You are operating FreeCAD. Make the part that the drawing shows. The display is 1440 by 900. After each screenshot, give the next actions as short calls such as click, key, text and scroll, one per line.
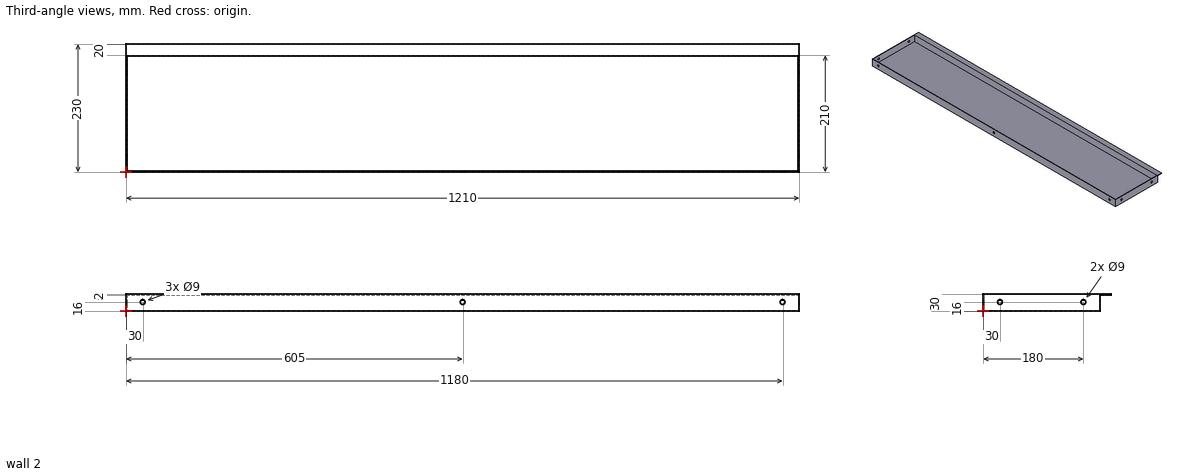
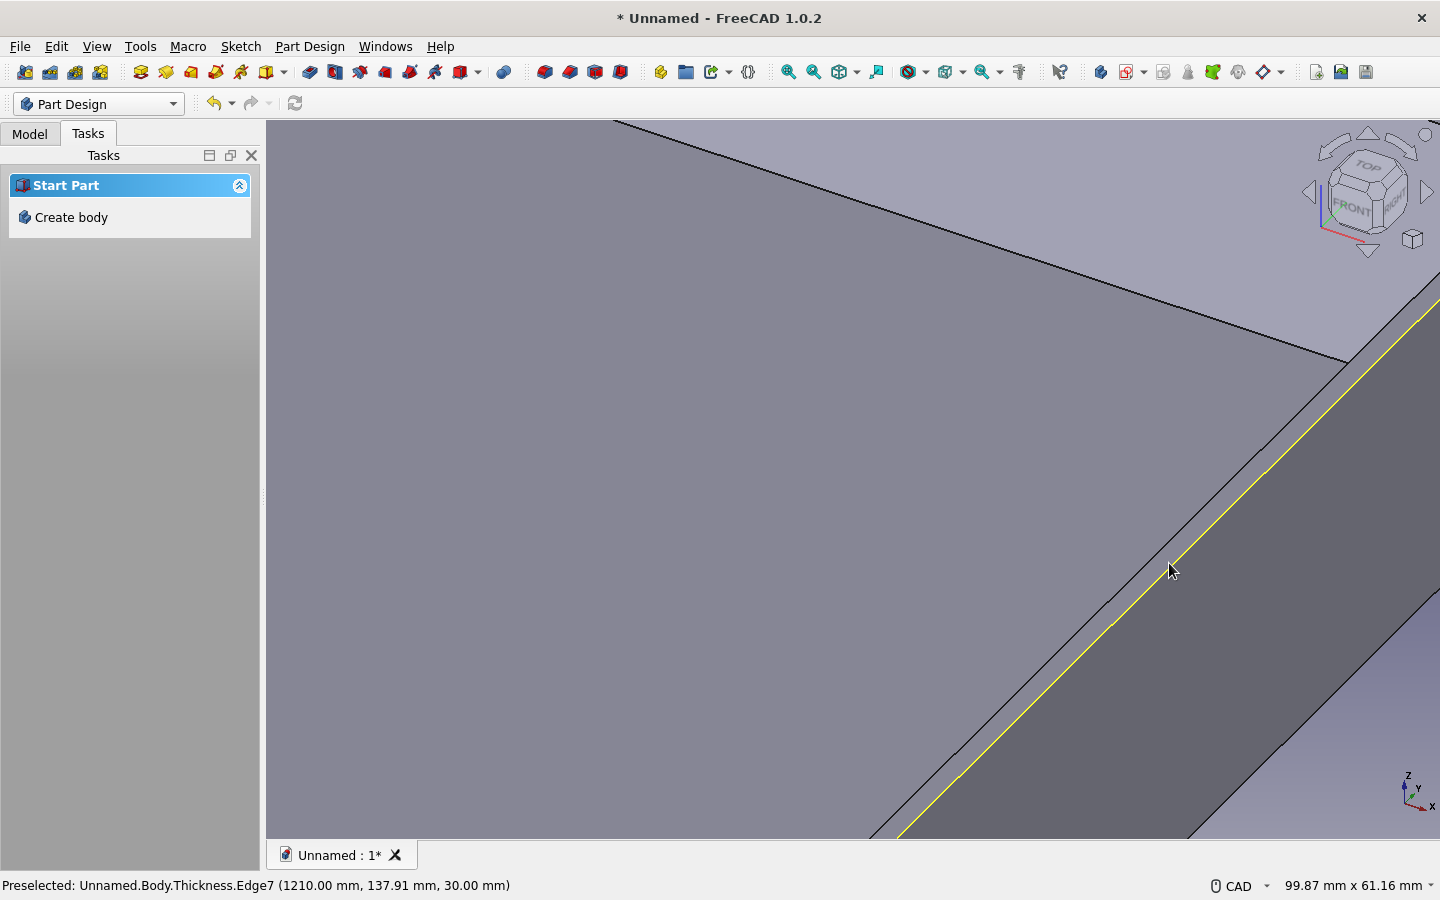
click(789, 72)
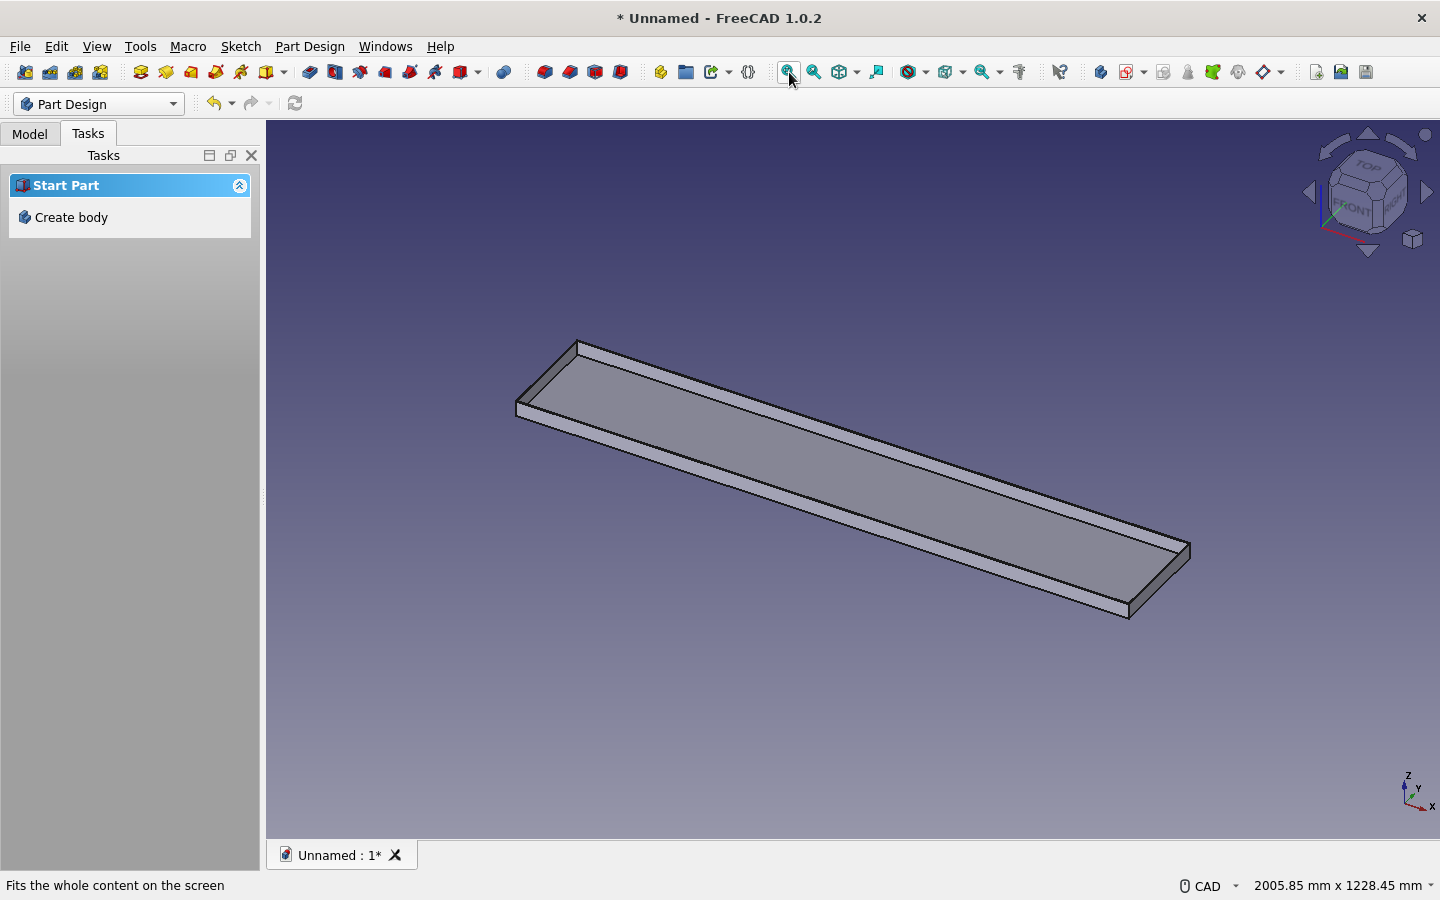
key(0)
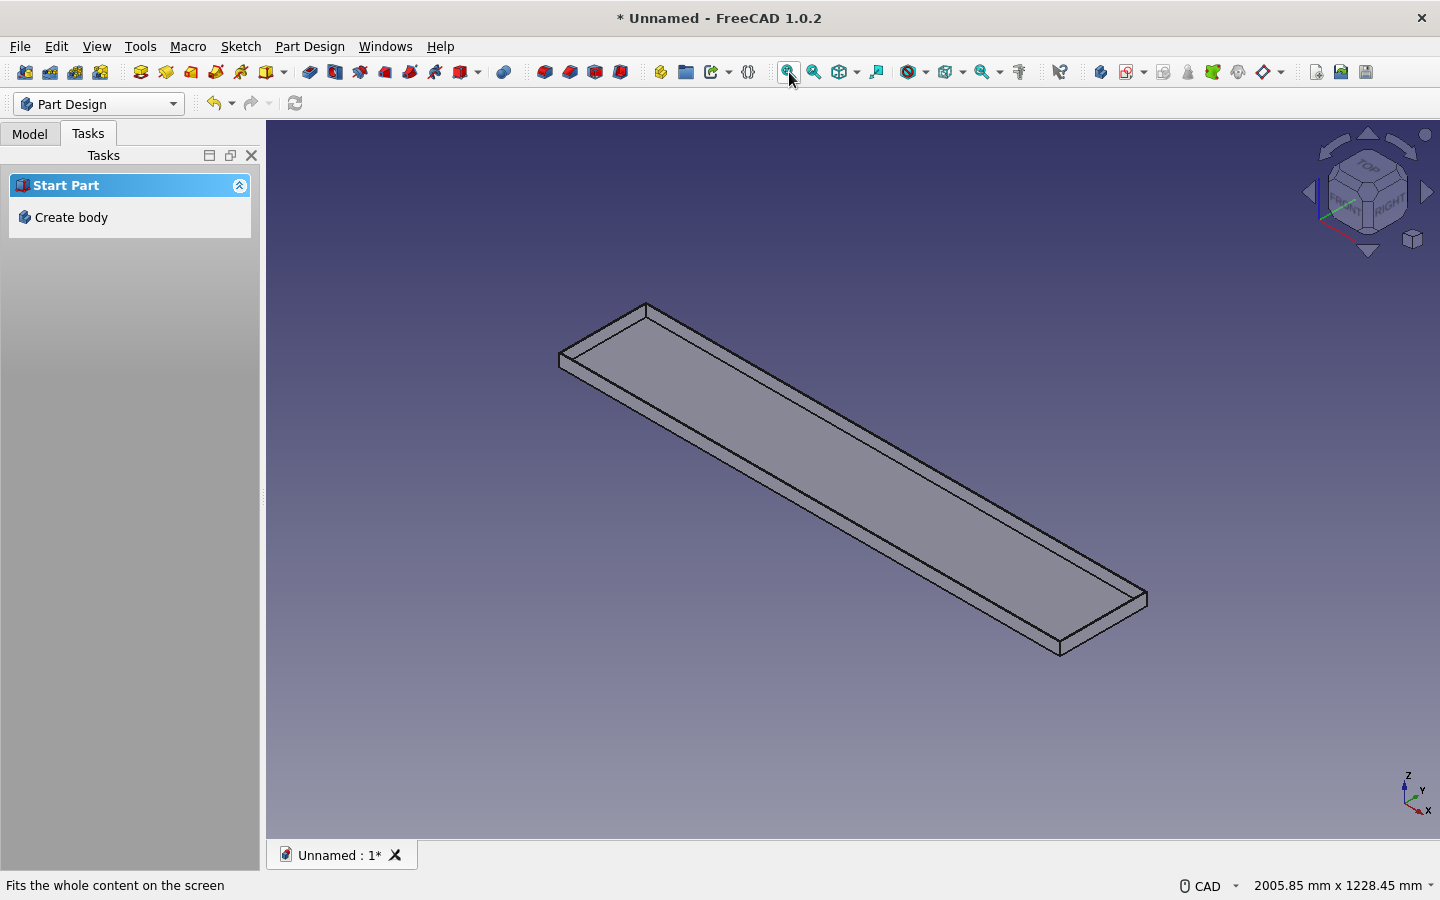
scroll(1117, 608, up, 15)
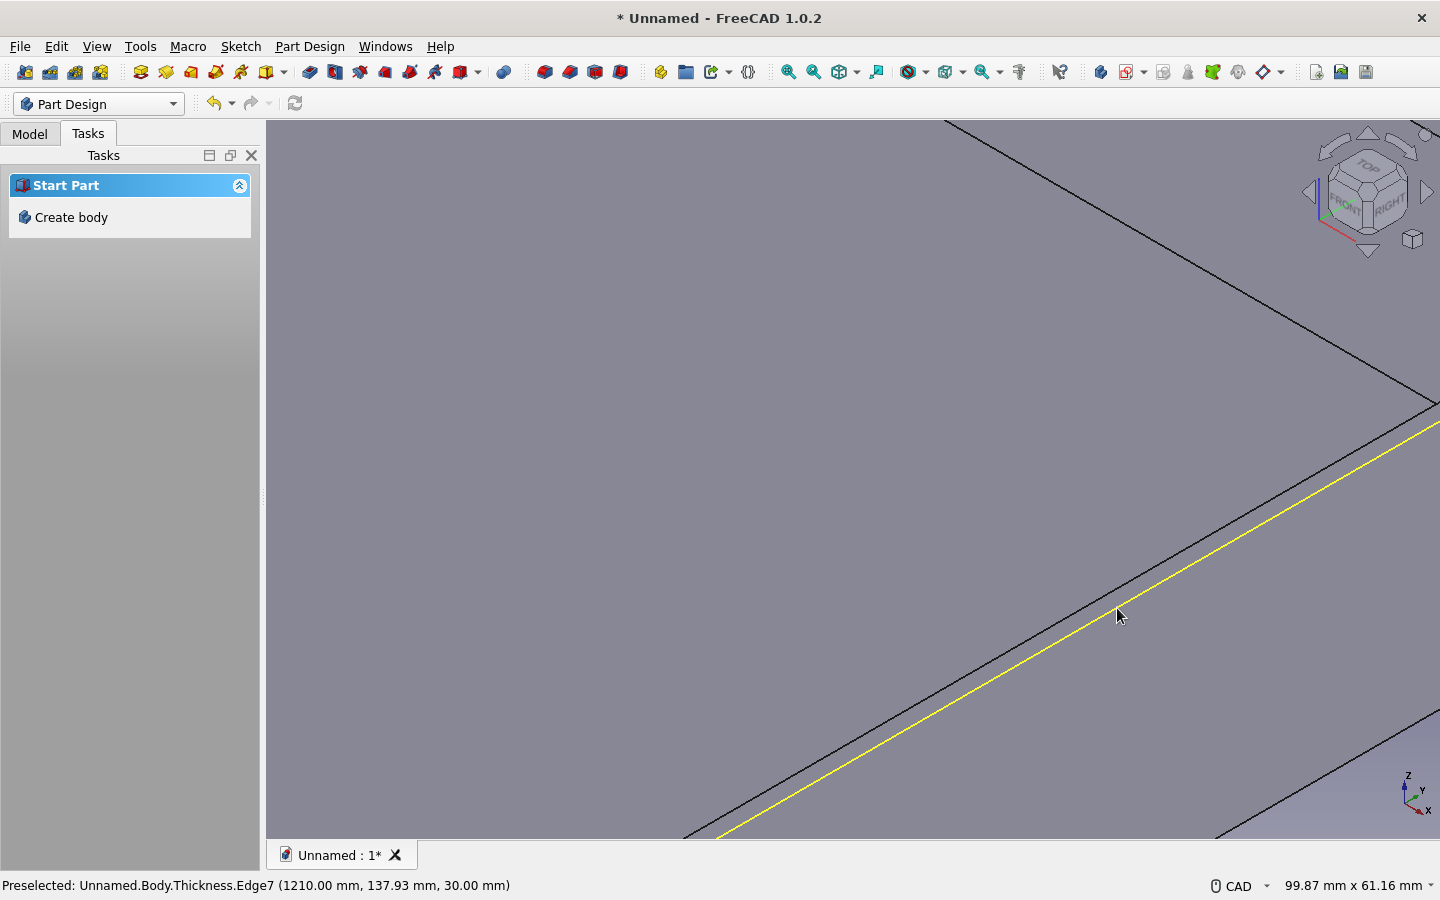
click(789, 72)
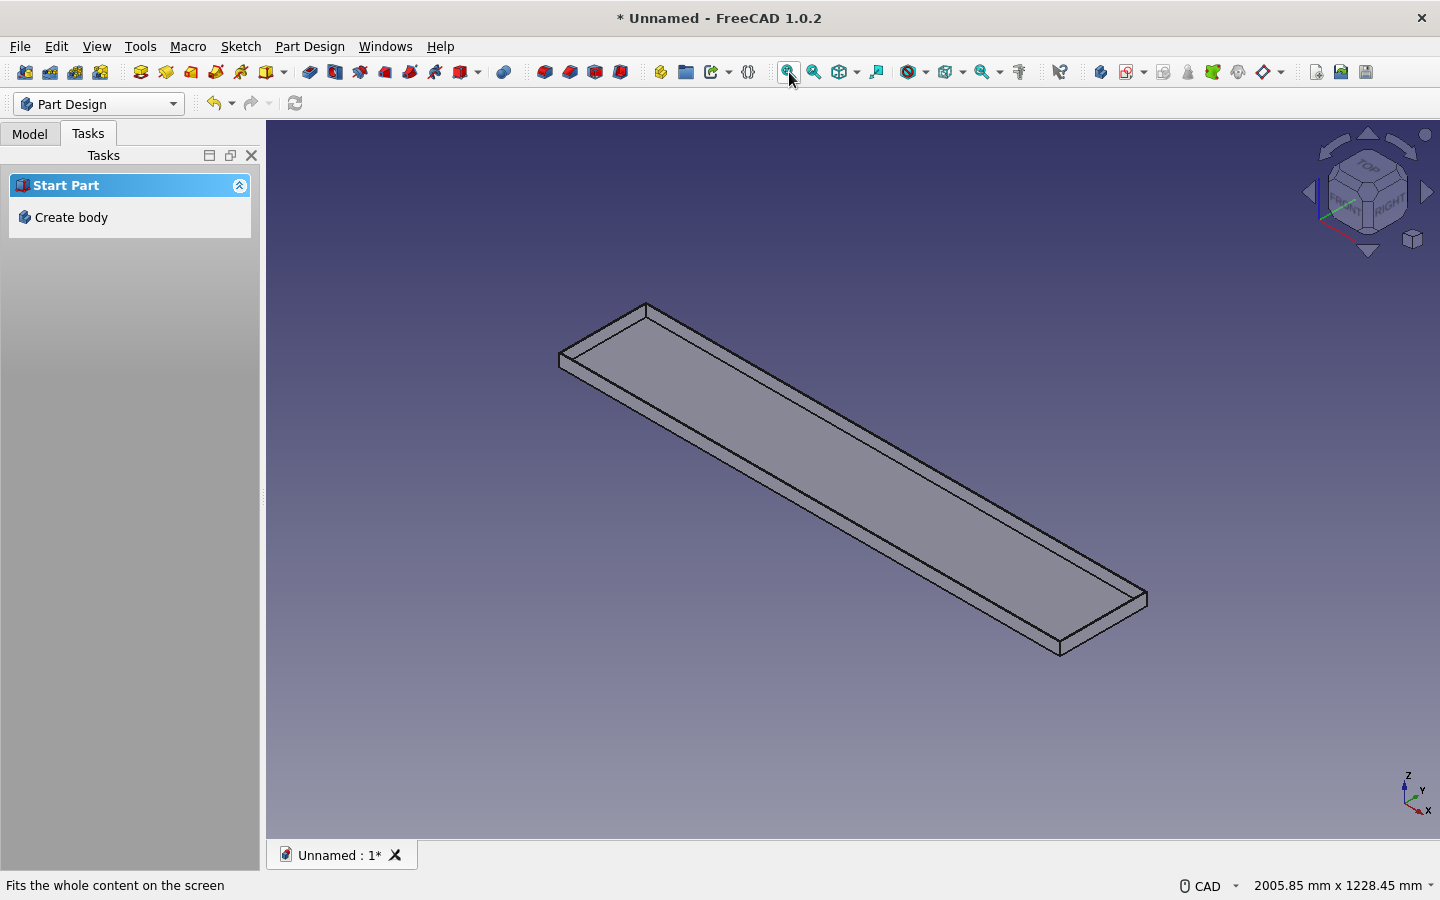
key(2)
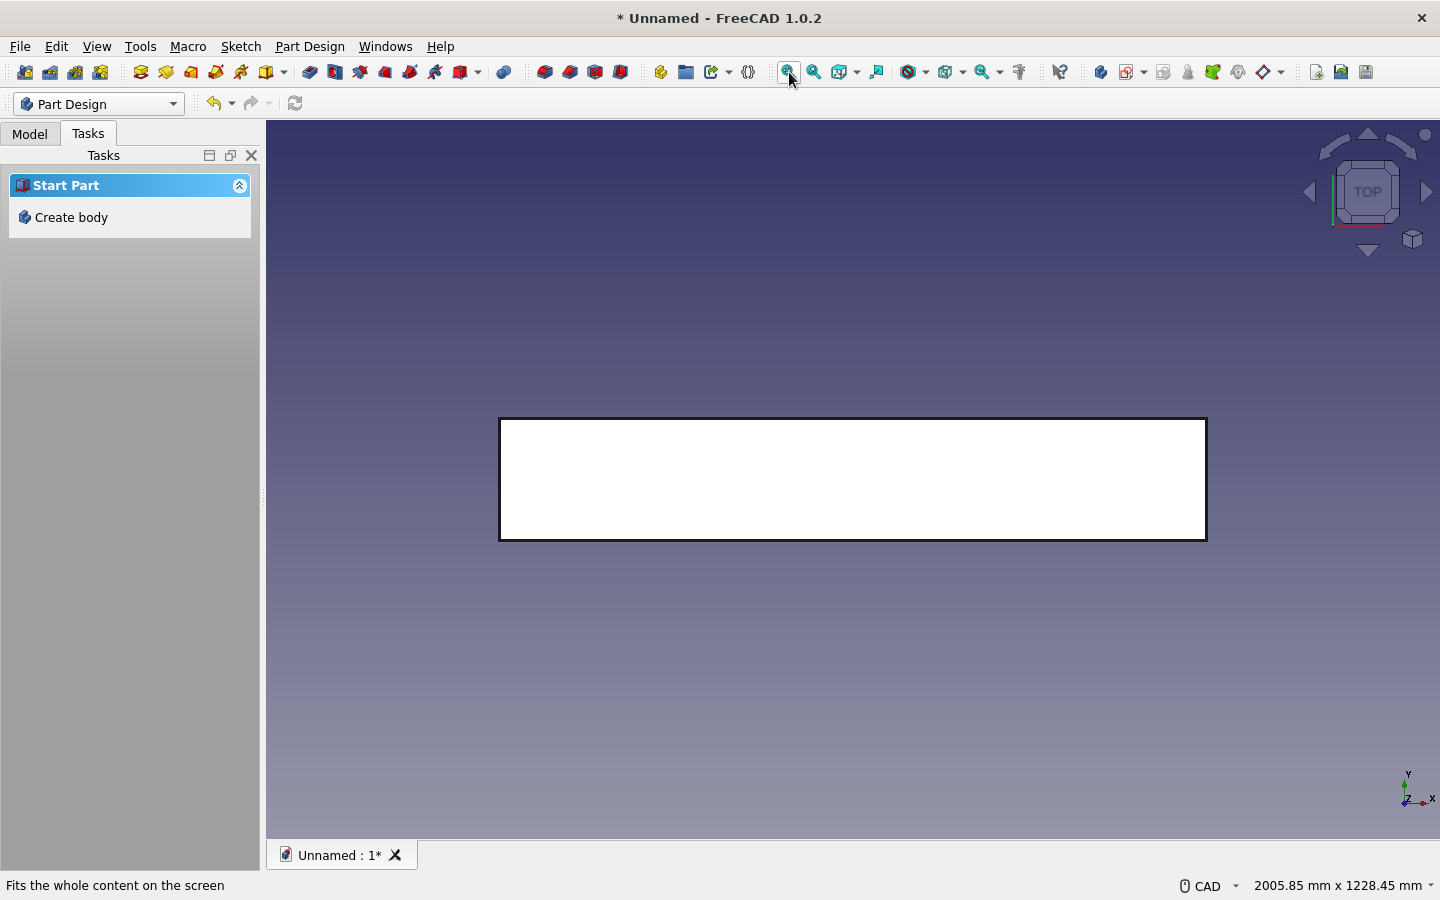
scroll(1207, 458, up, 15)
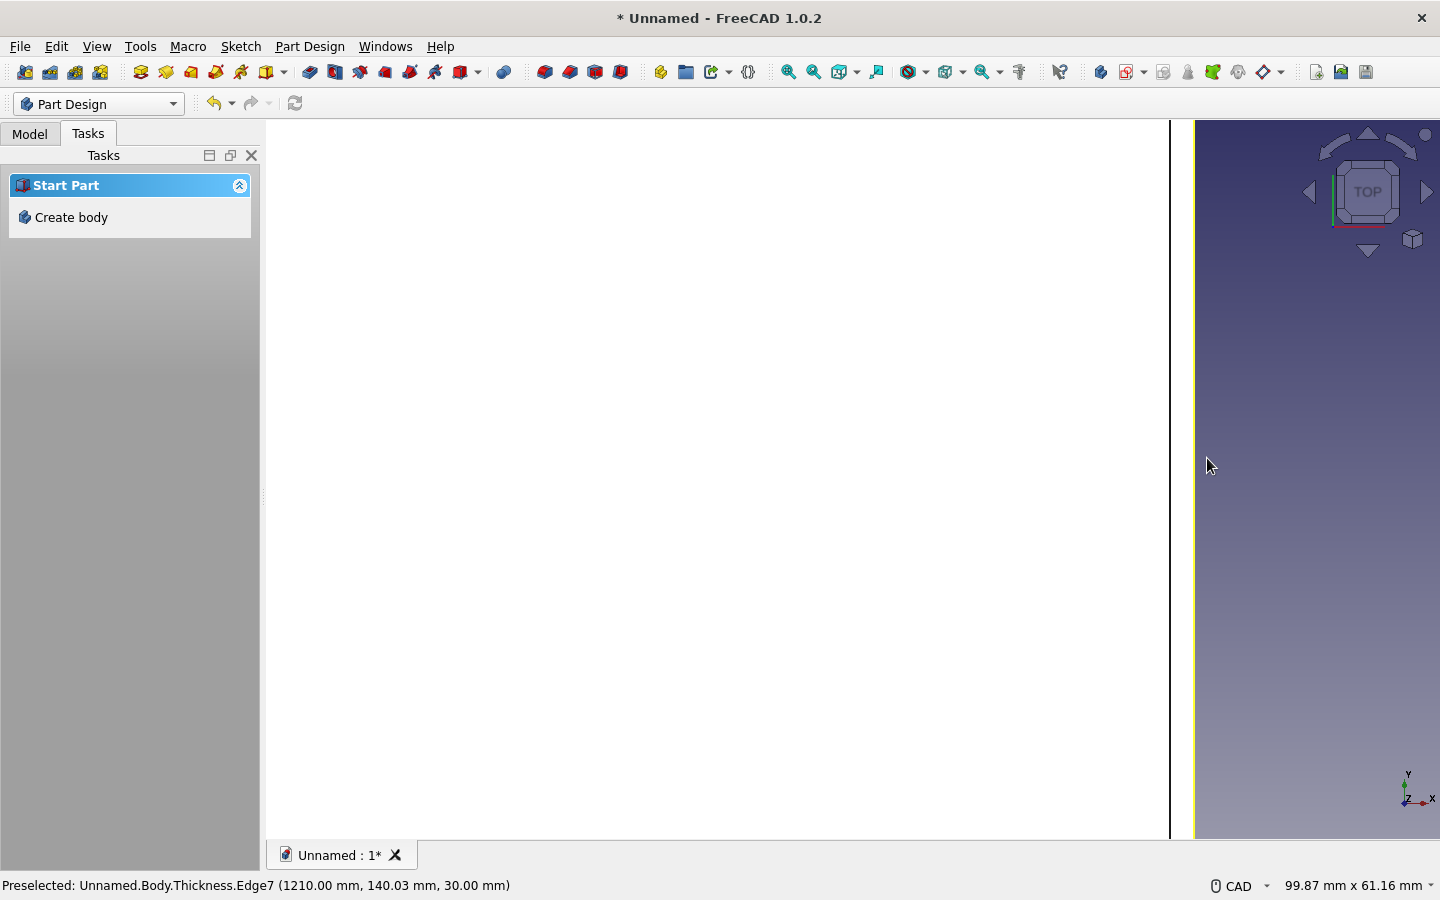
click(789, 72)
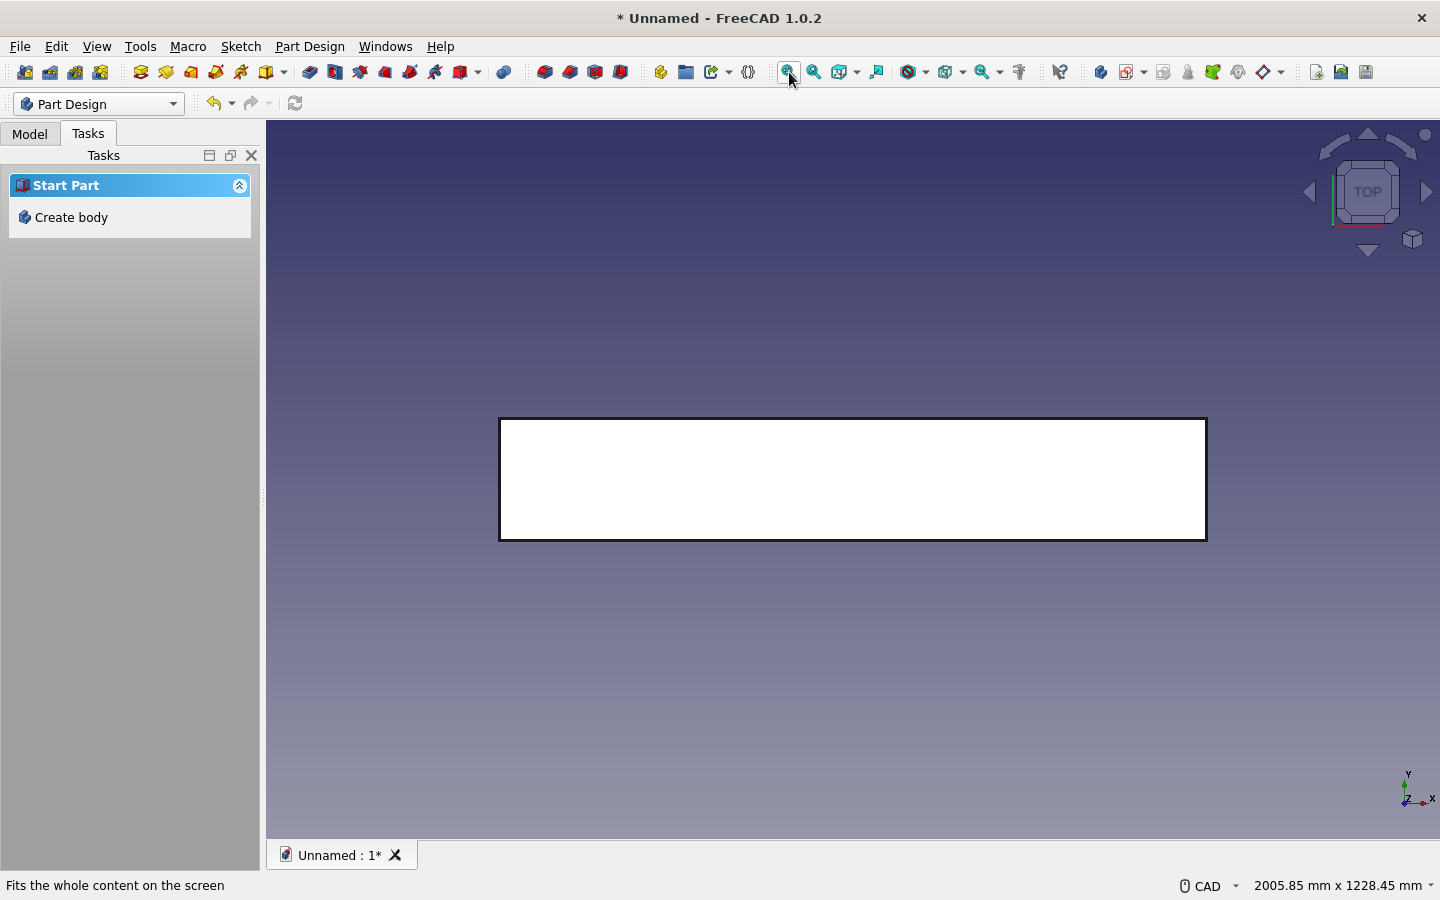
key(1)